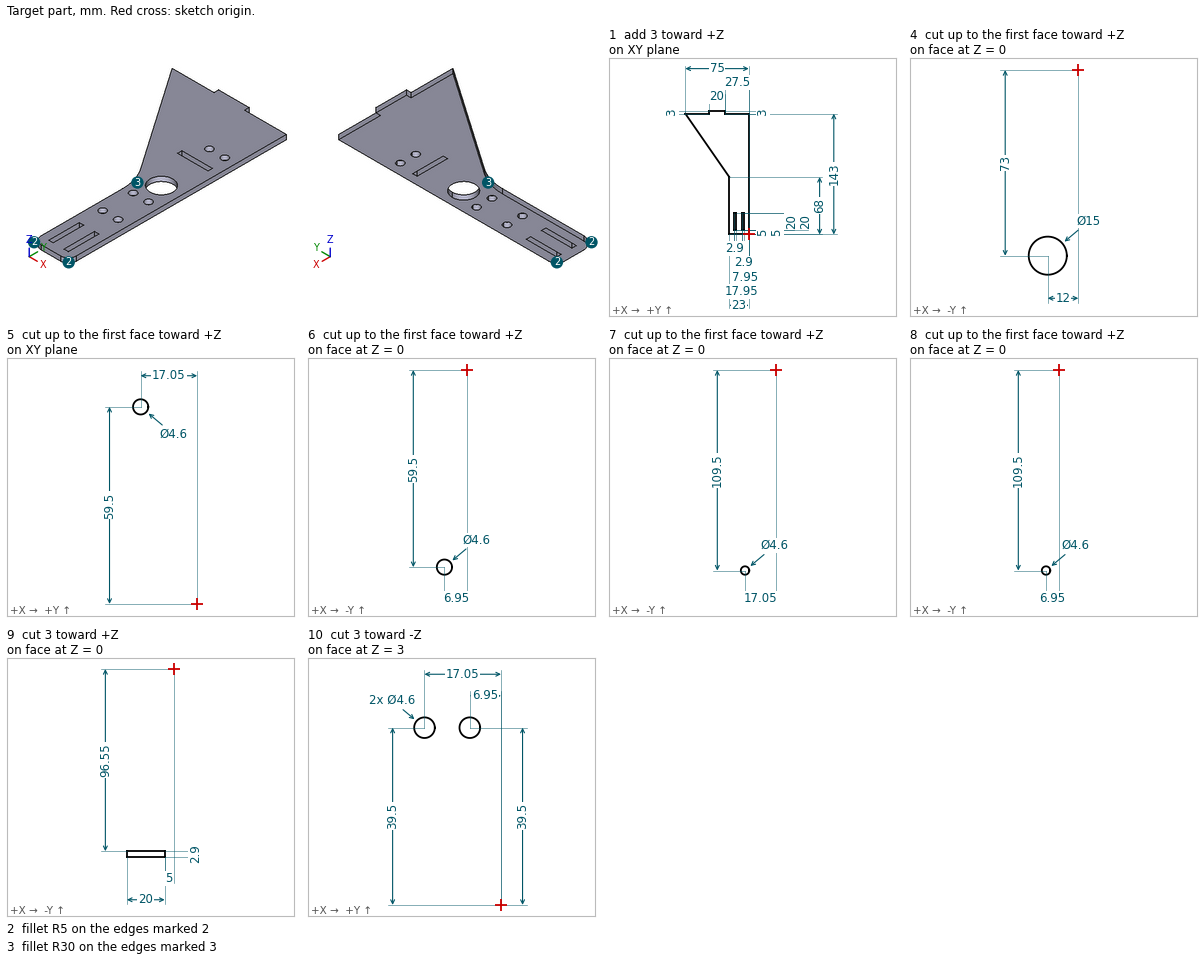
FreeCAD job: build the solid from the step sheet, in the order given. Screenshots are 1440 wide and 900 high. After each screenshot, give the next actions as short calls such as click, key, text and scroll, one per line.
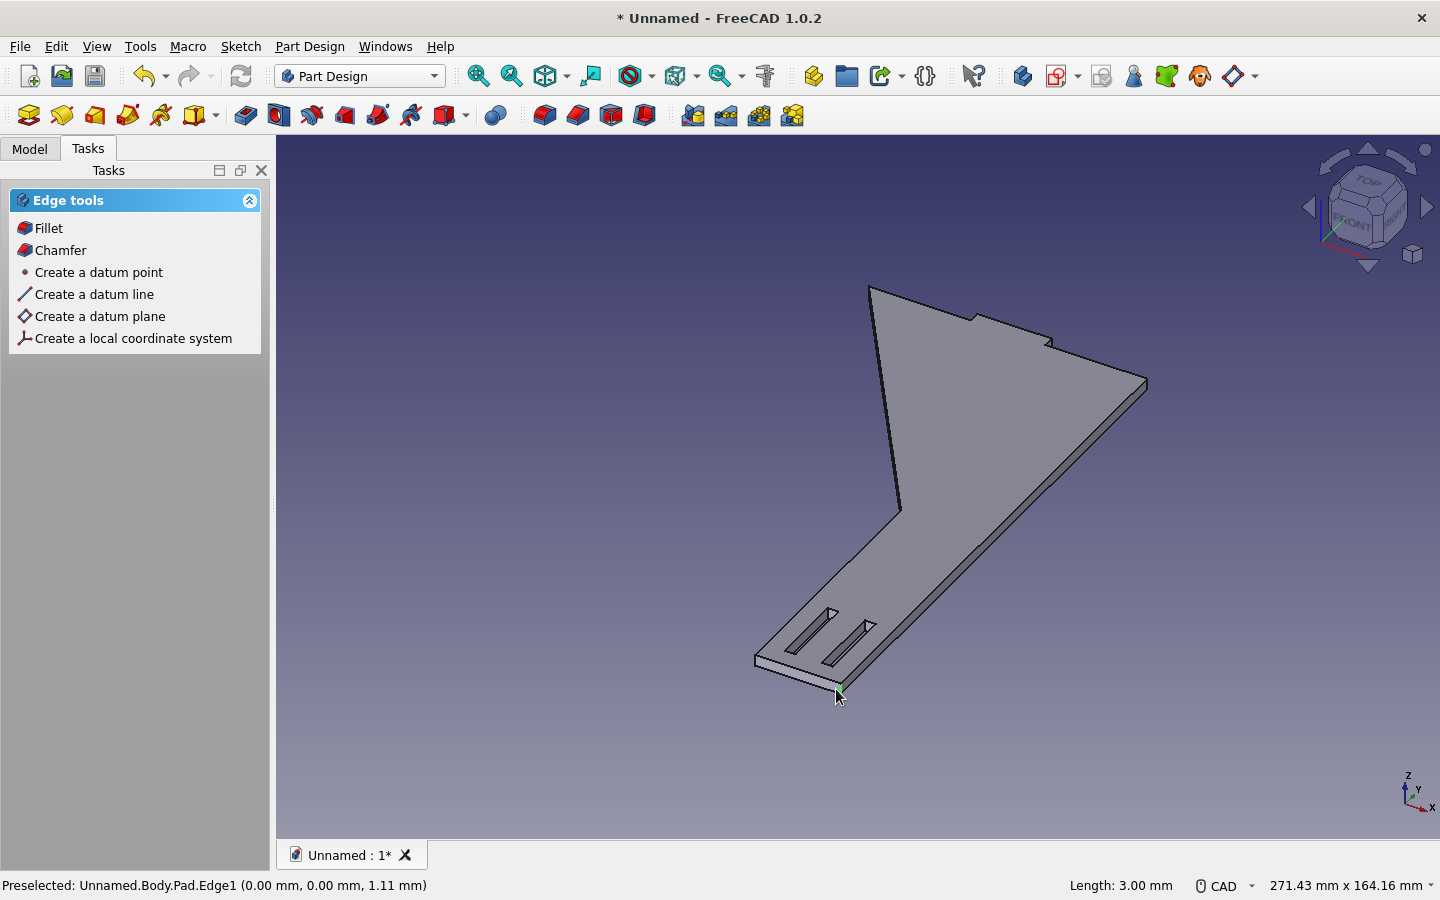
scroll(755, 659, up, 6)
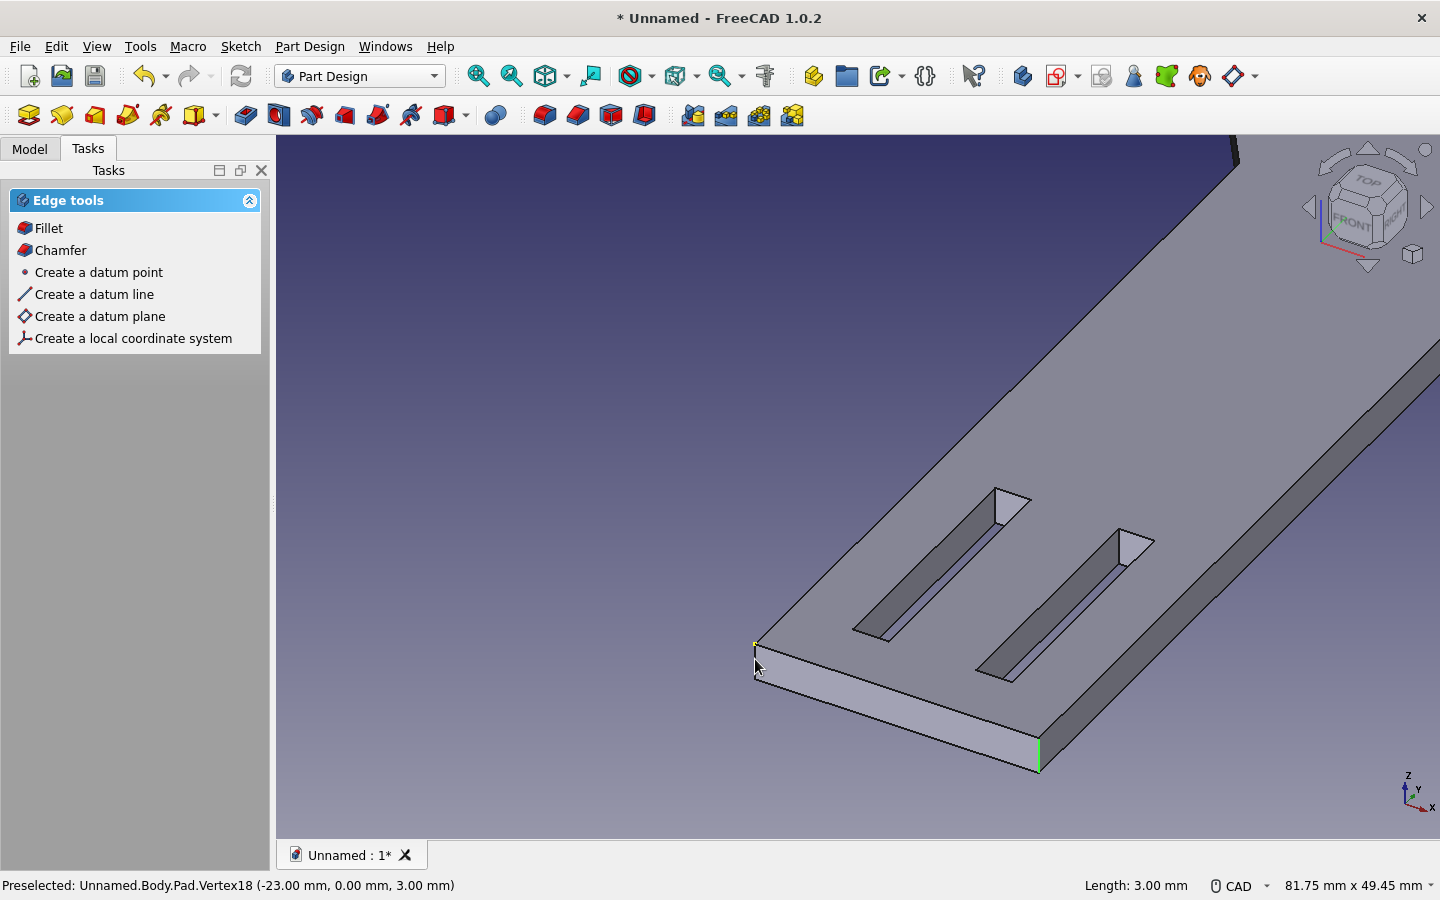
click(479, 76)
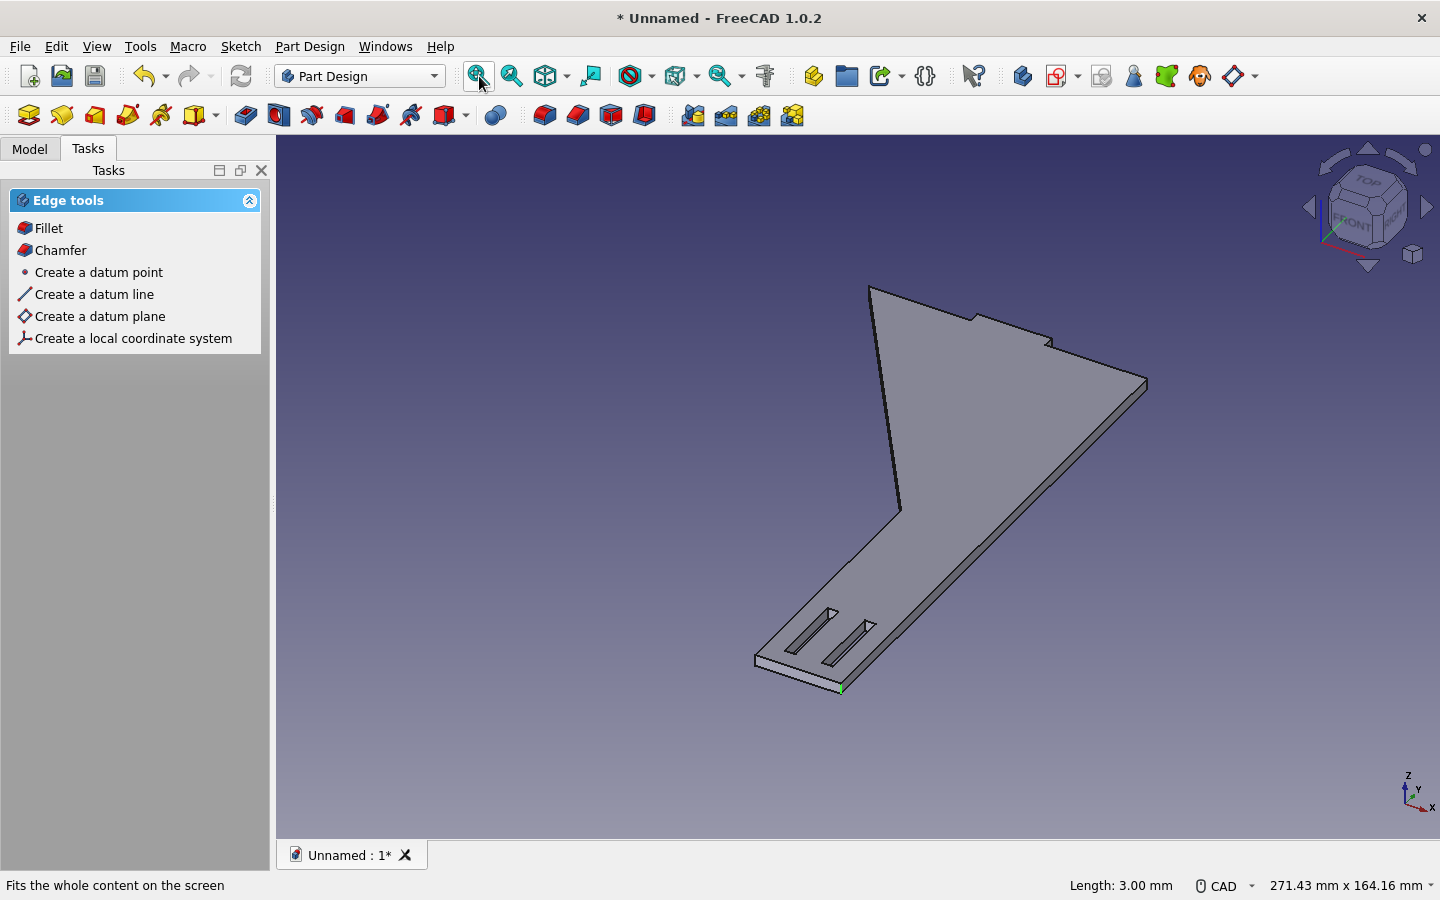
key(0)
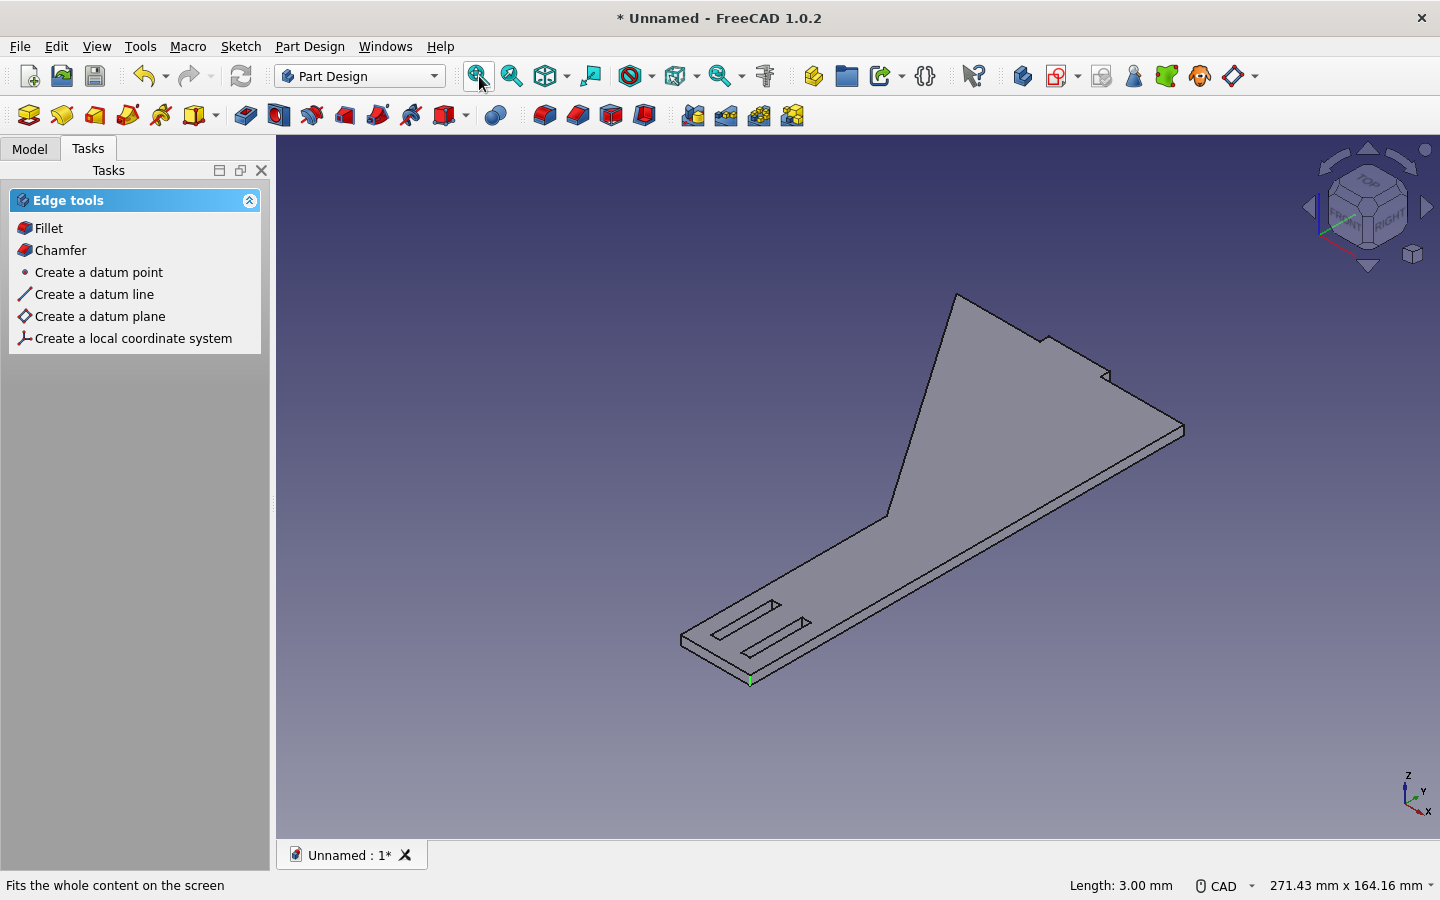
scroll(681, 639, up, 6)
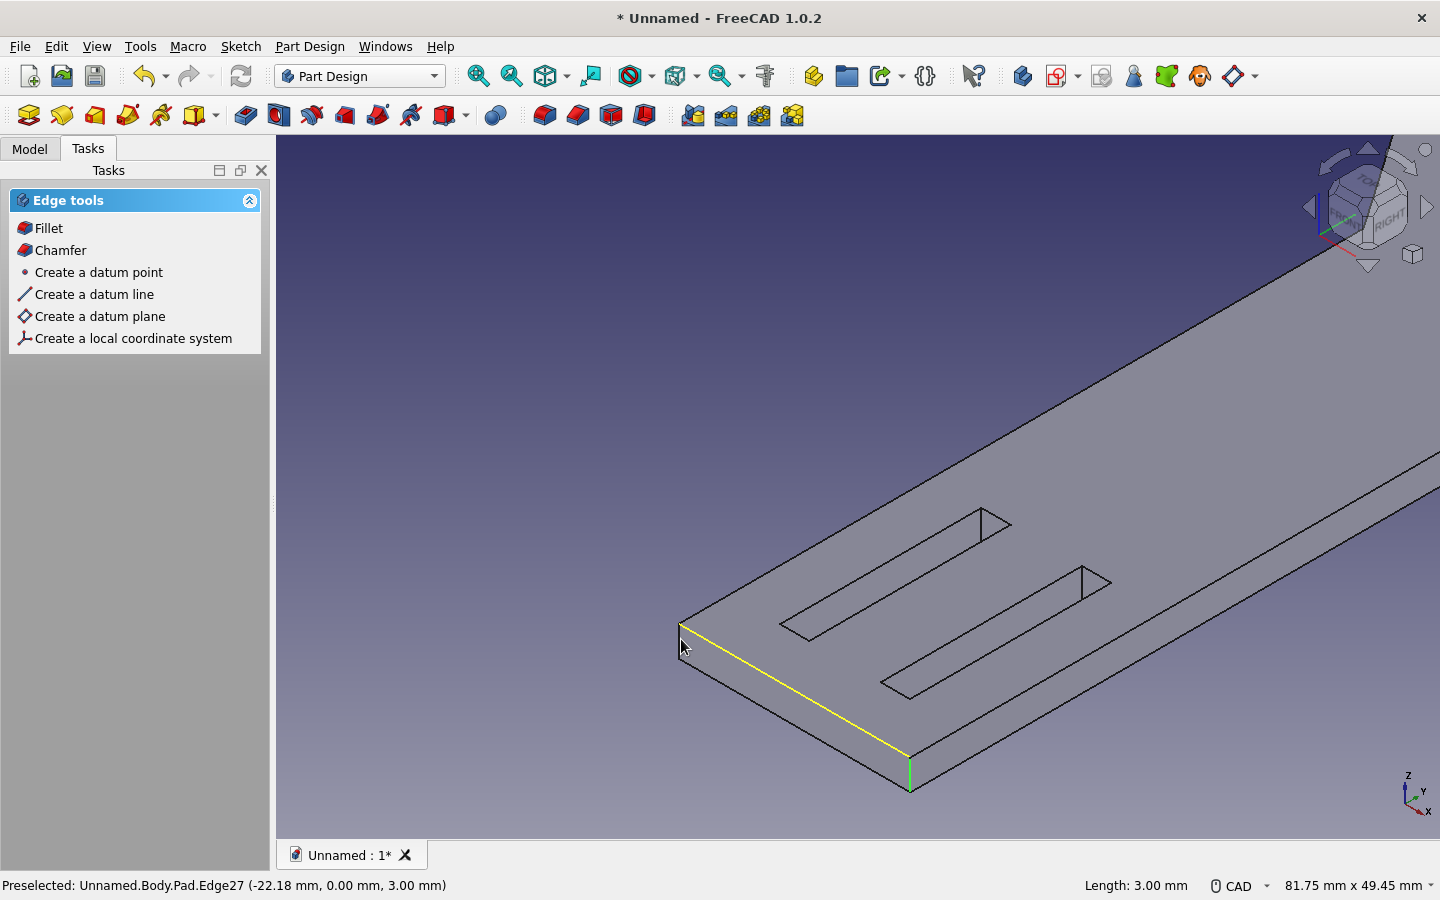
key(v)
key(f)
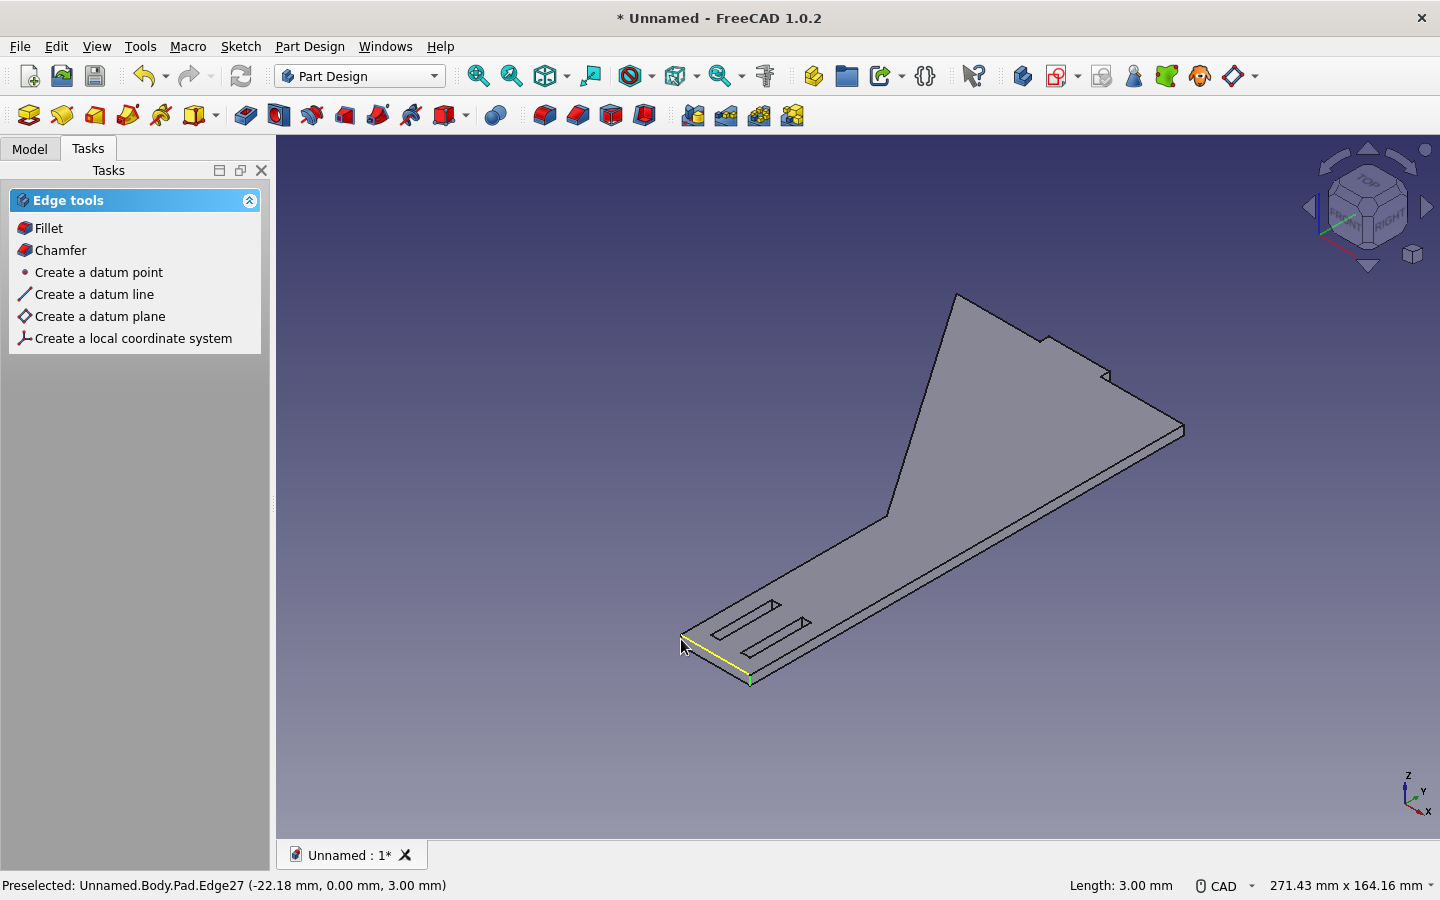
key(2)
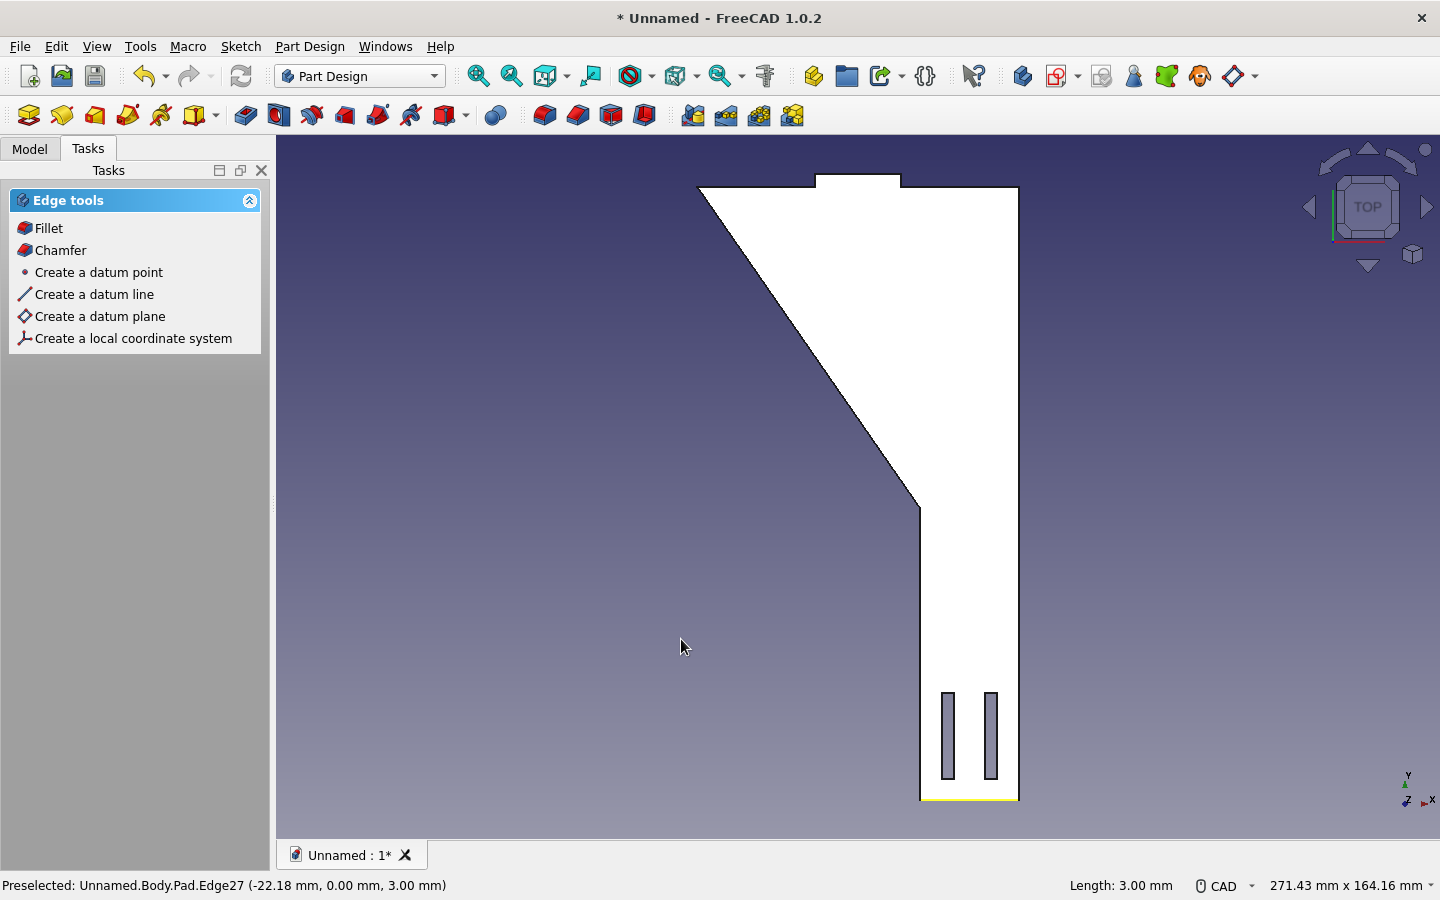
scroll(920, 799, up, 6)